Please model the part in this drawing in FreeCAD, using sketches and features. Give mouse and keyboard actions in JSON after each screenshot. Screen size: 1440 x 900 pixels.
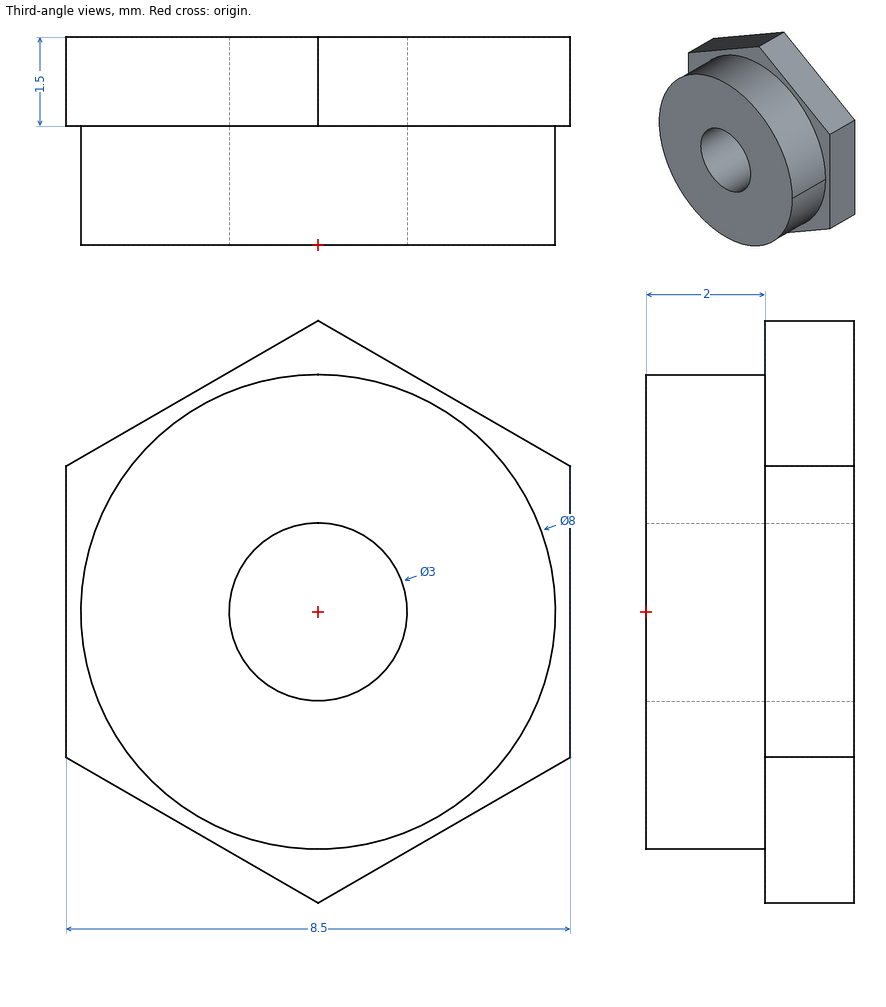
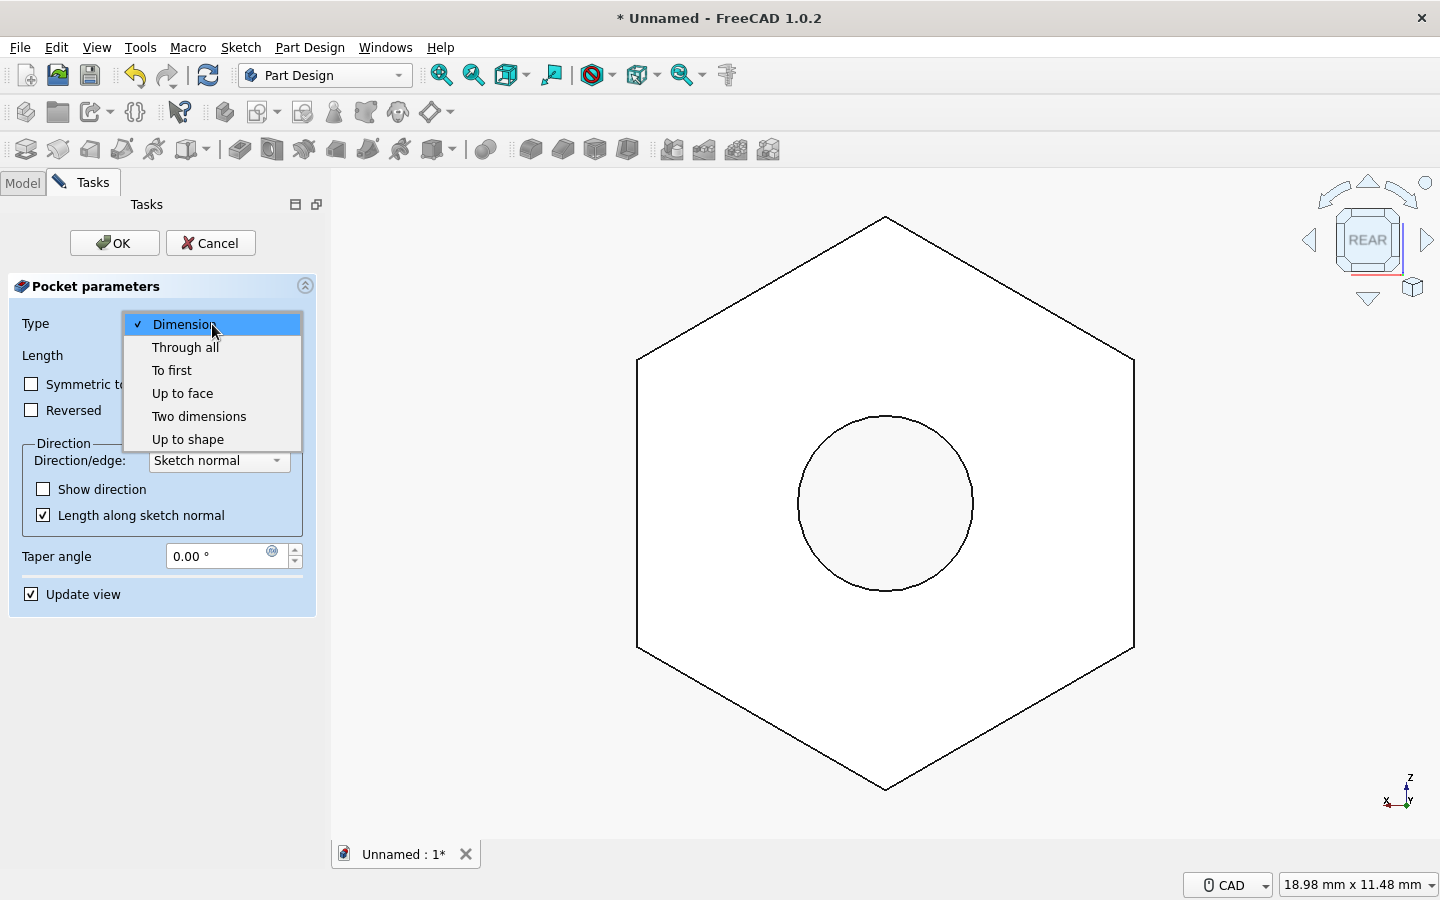
{"action": "left_click", "coordinate": [212, 348]}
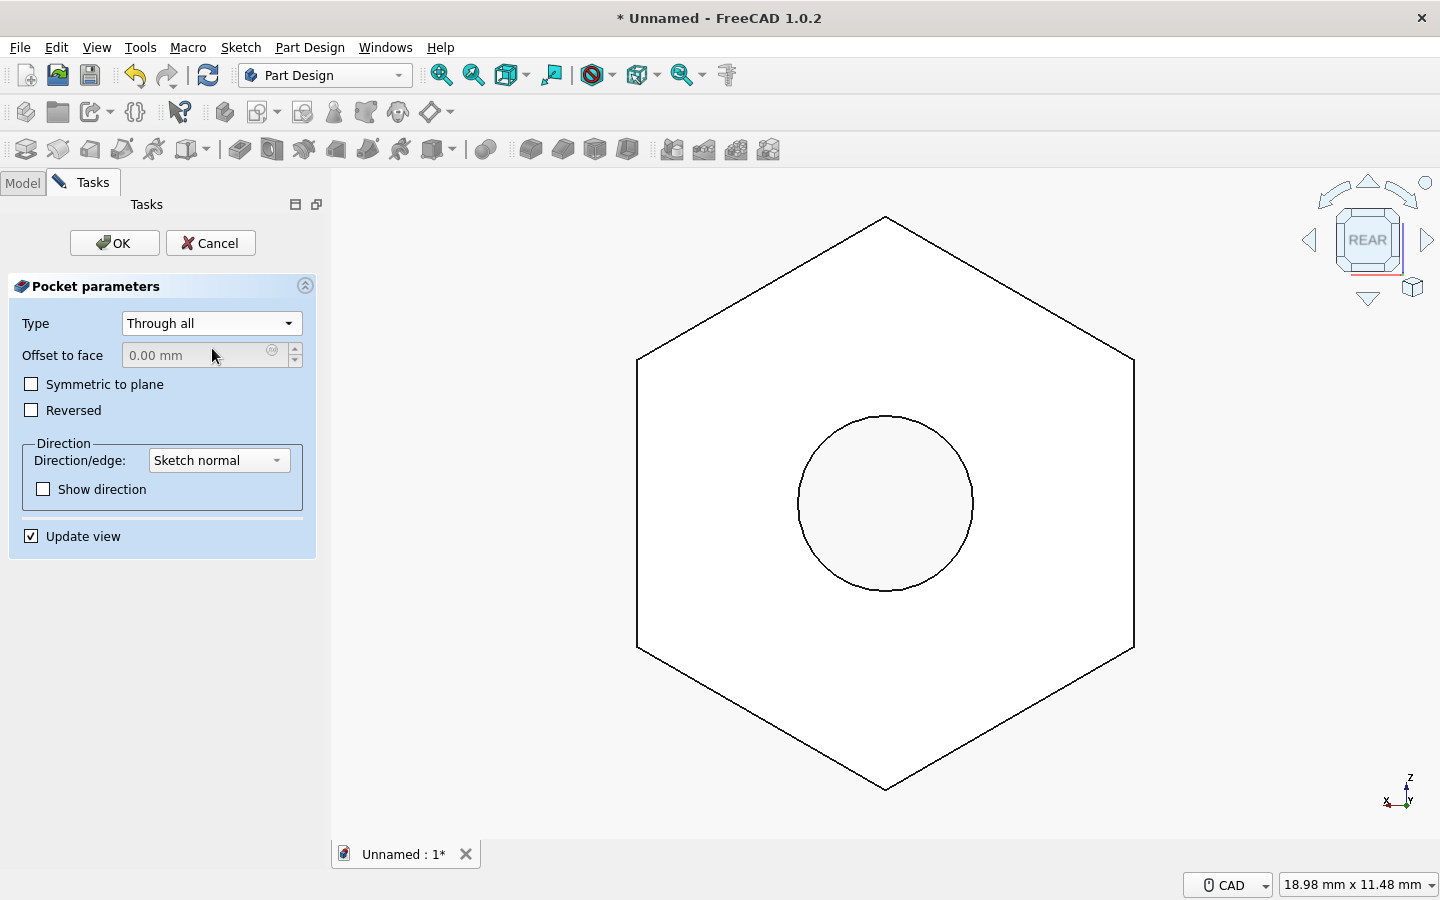
{"action": "left_click", "coordinate": [115, 243]}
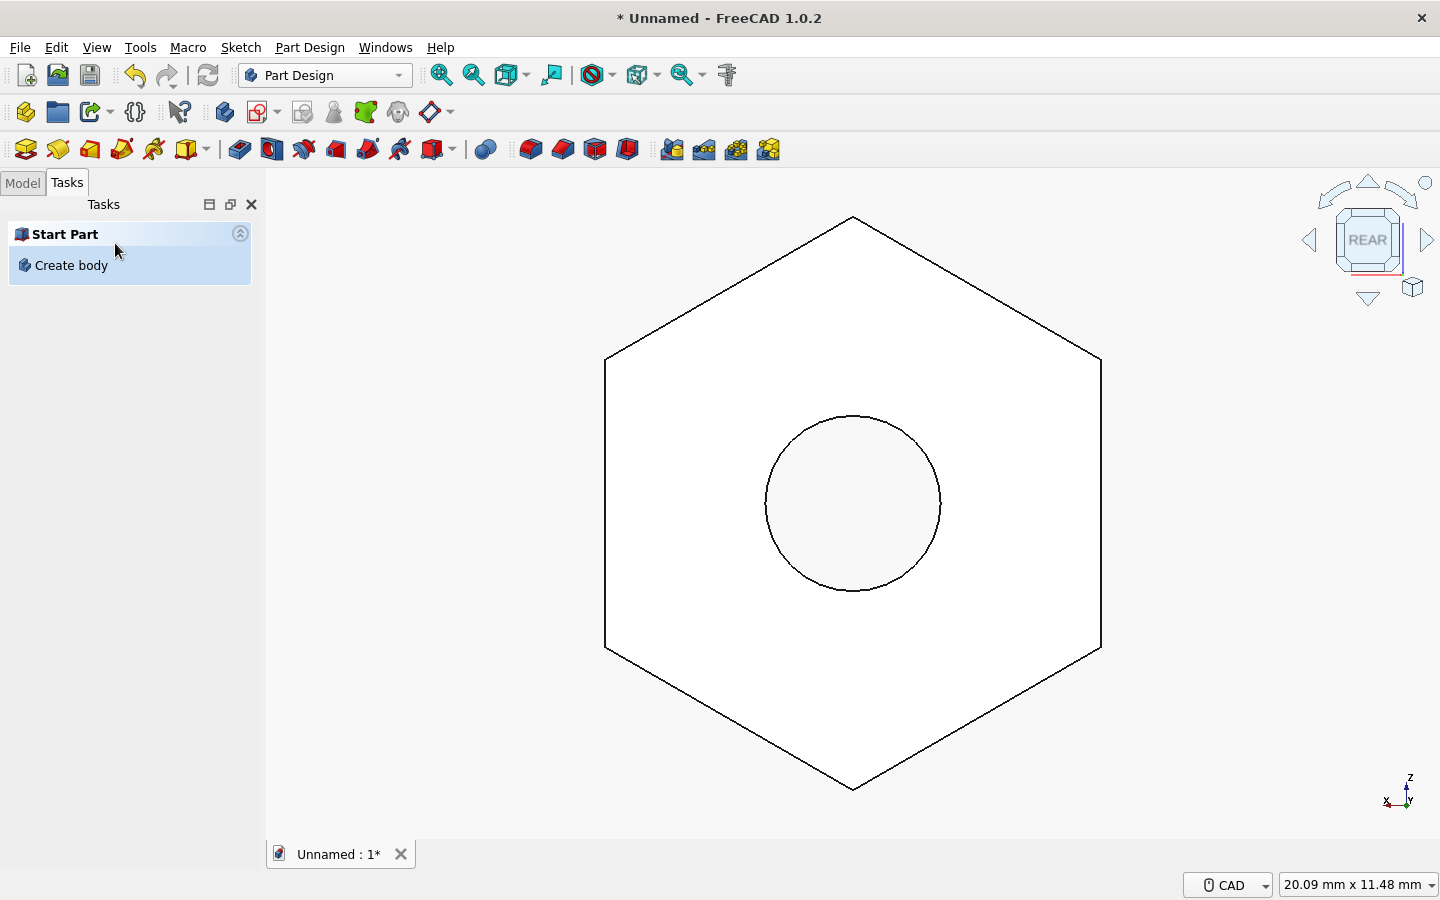
{"action": "key", "text": "0"}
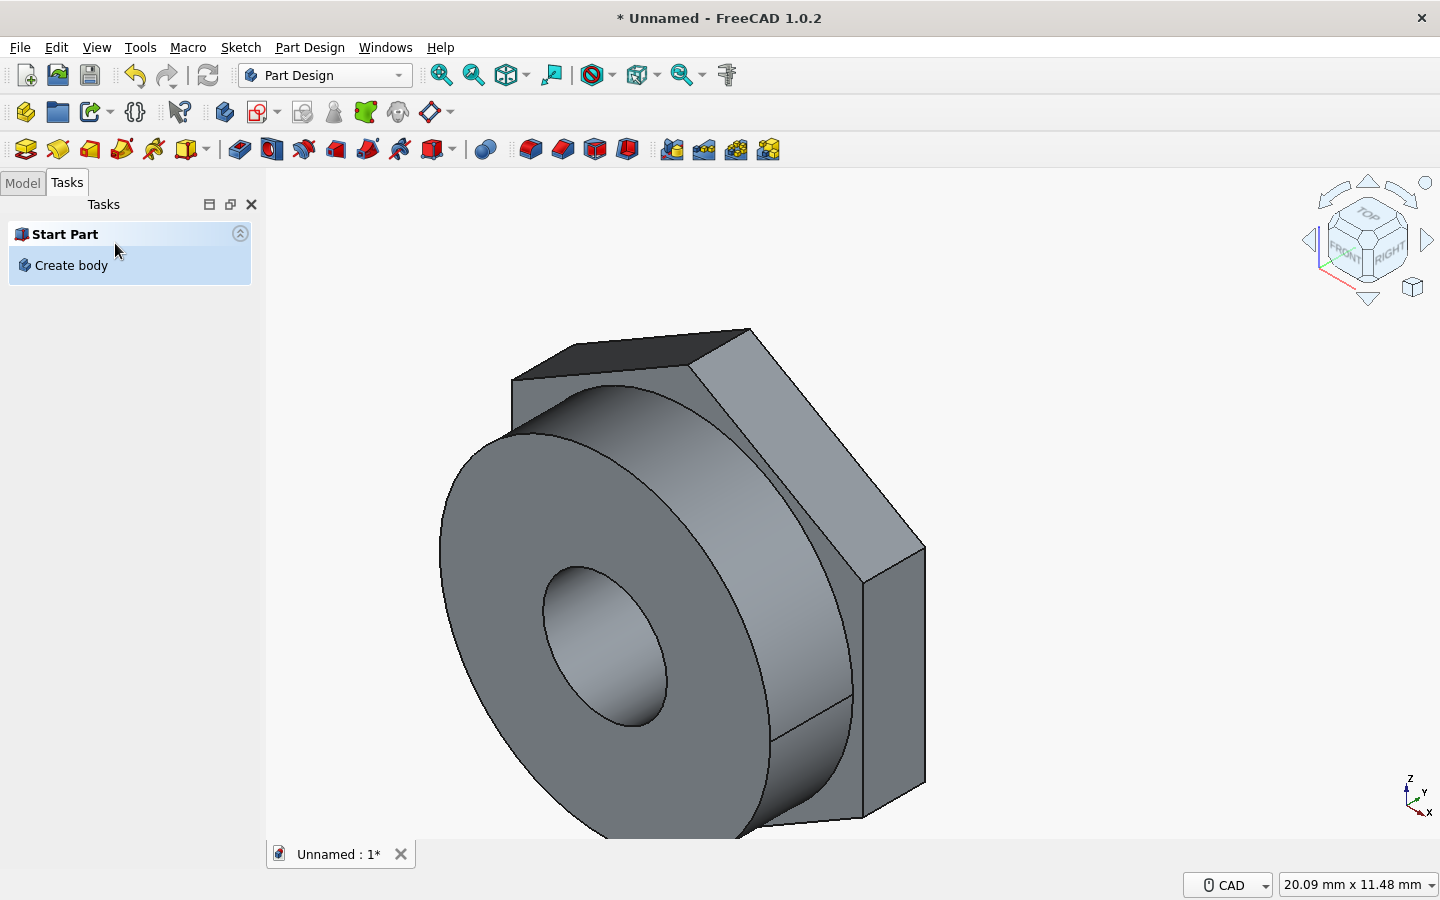
{"action": "key", "text": "v f"}